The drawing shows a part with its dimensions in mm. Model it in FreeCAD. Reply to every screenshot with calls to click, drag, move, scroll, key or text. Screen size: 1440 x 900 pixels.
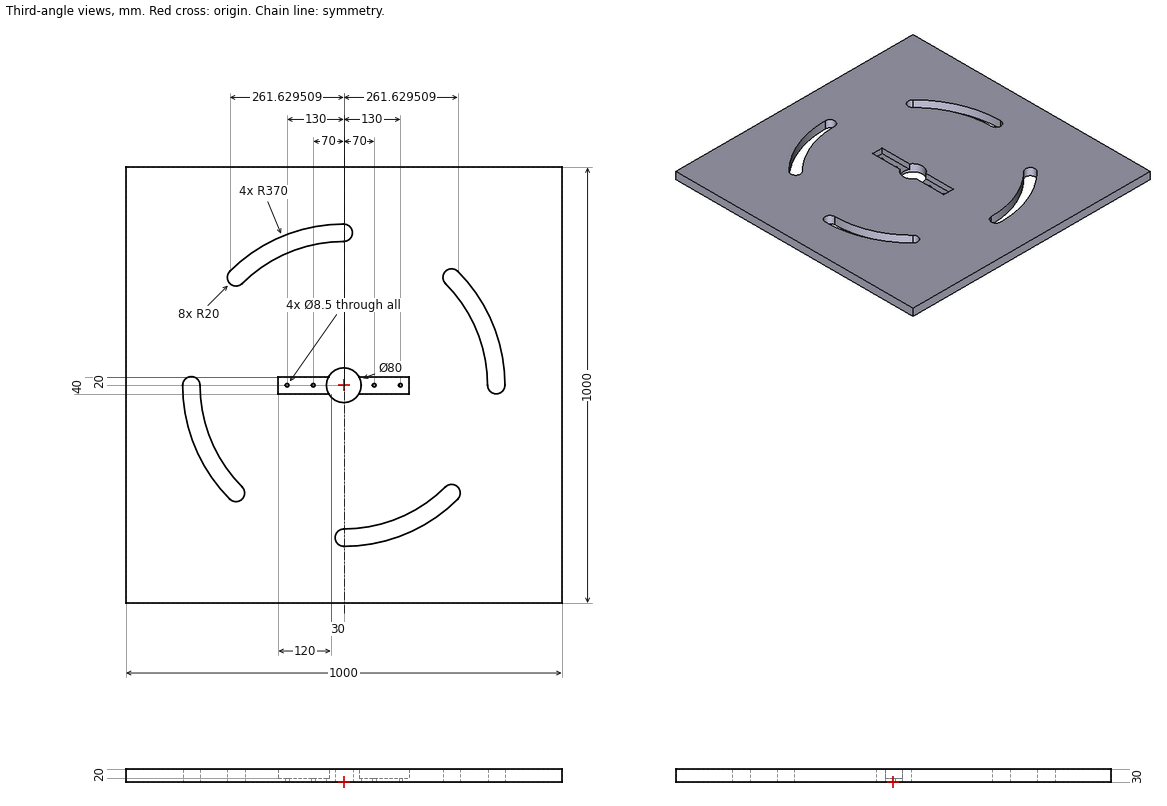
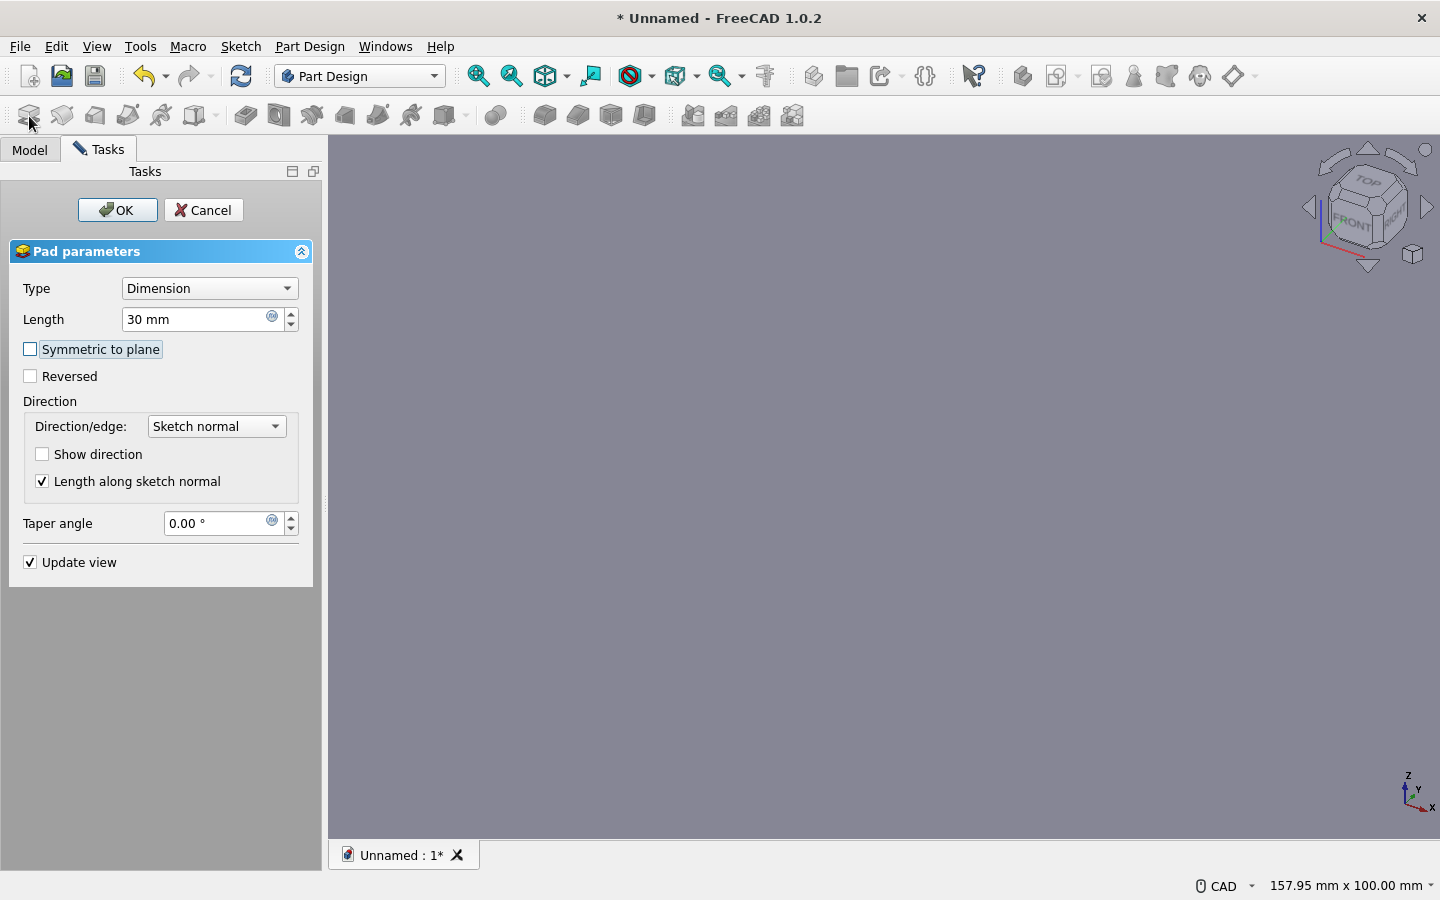
click(118, 210)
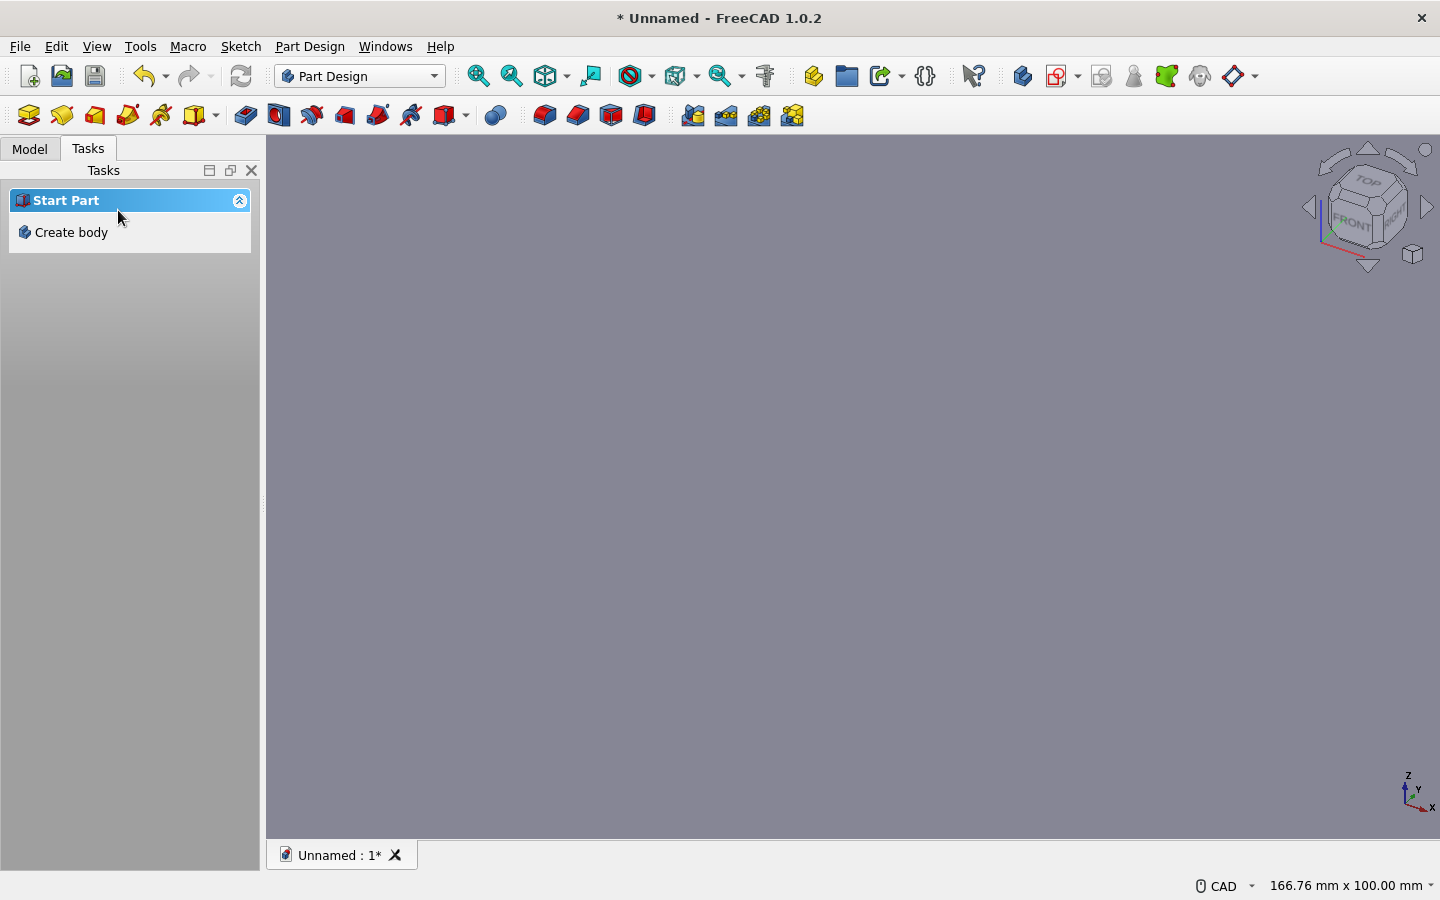
key(v)
key(f)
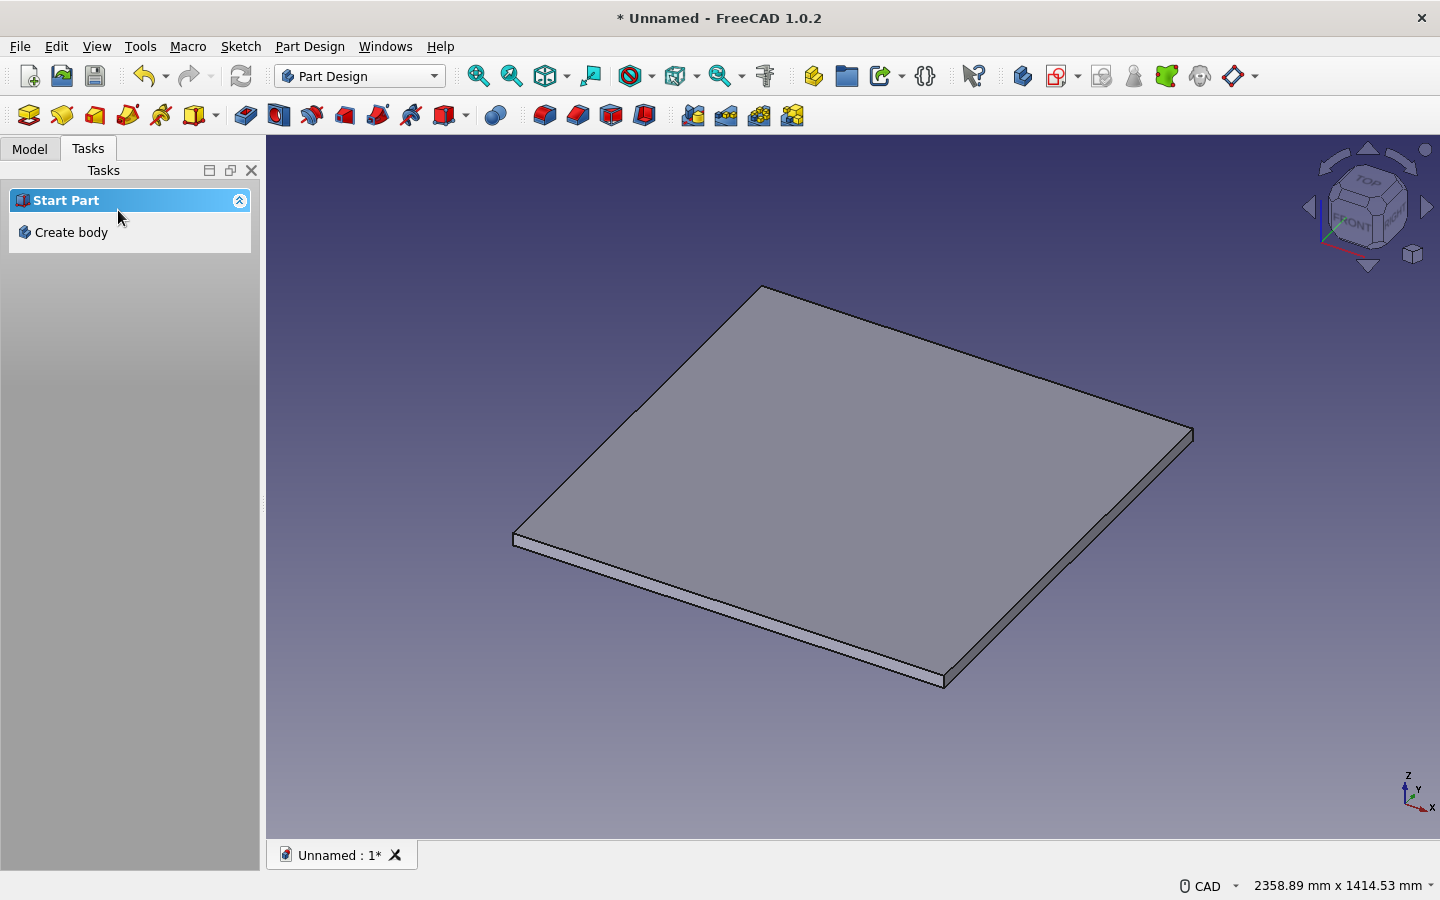
click(853, 480)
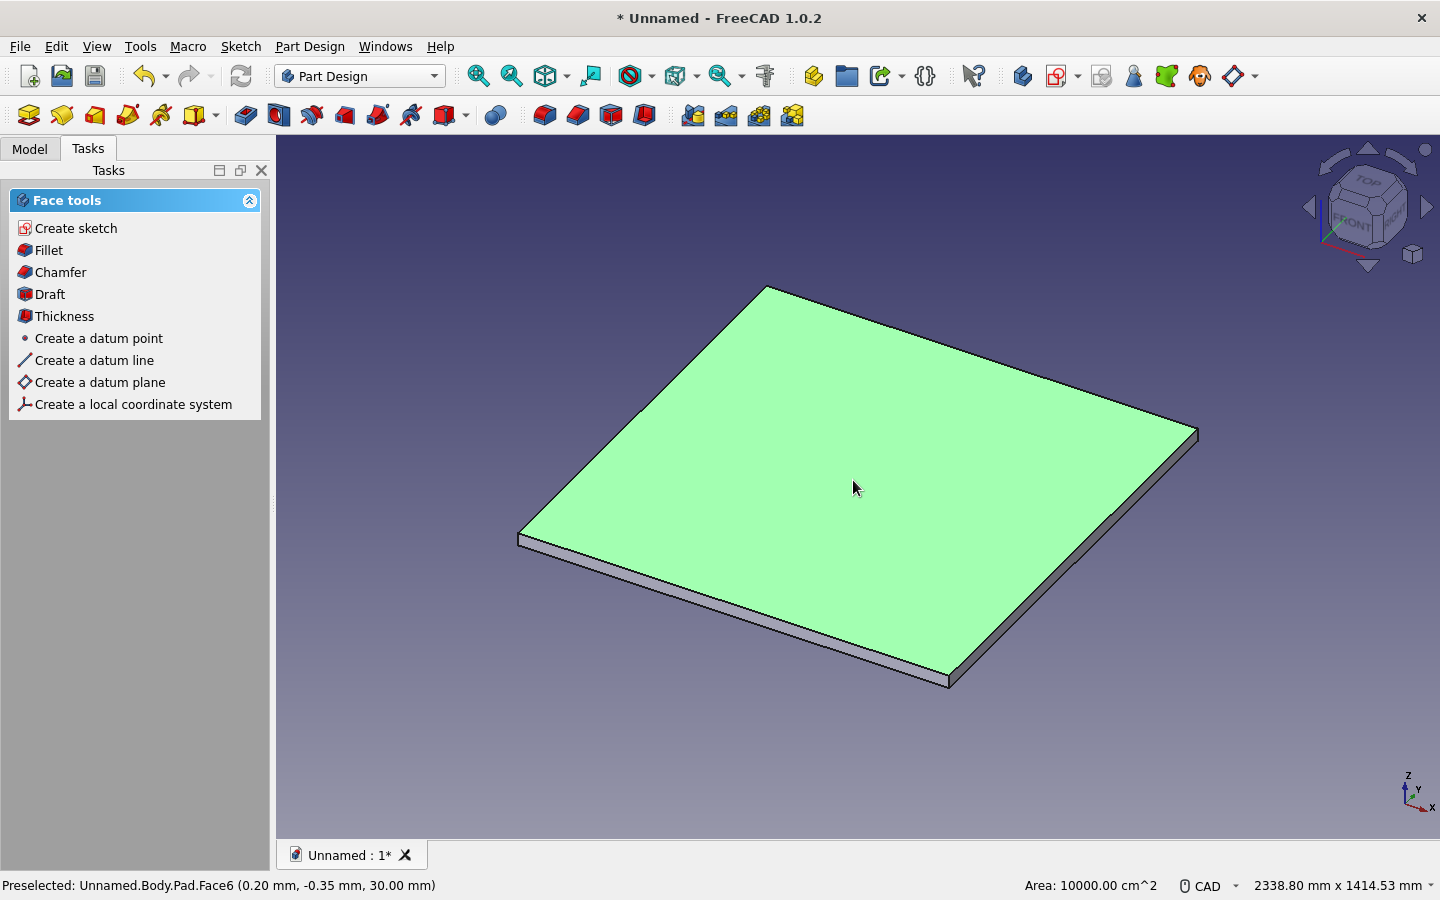
click(1056, 76)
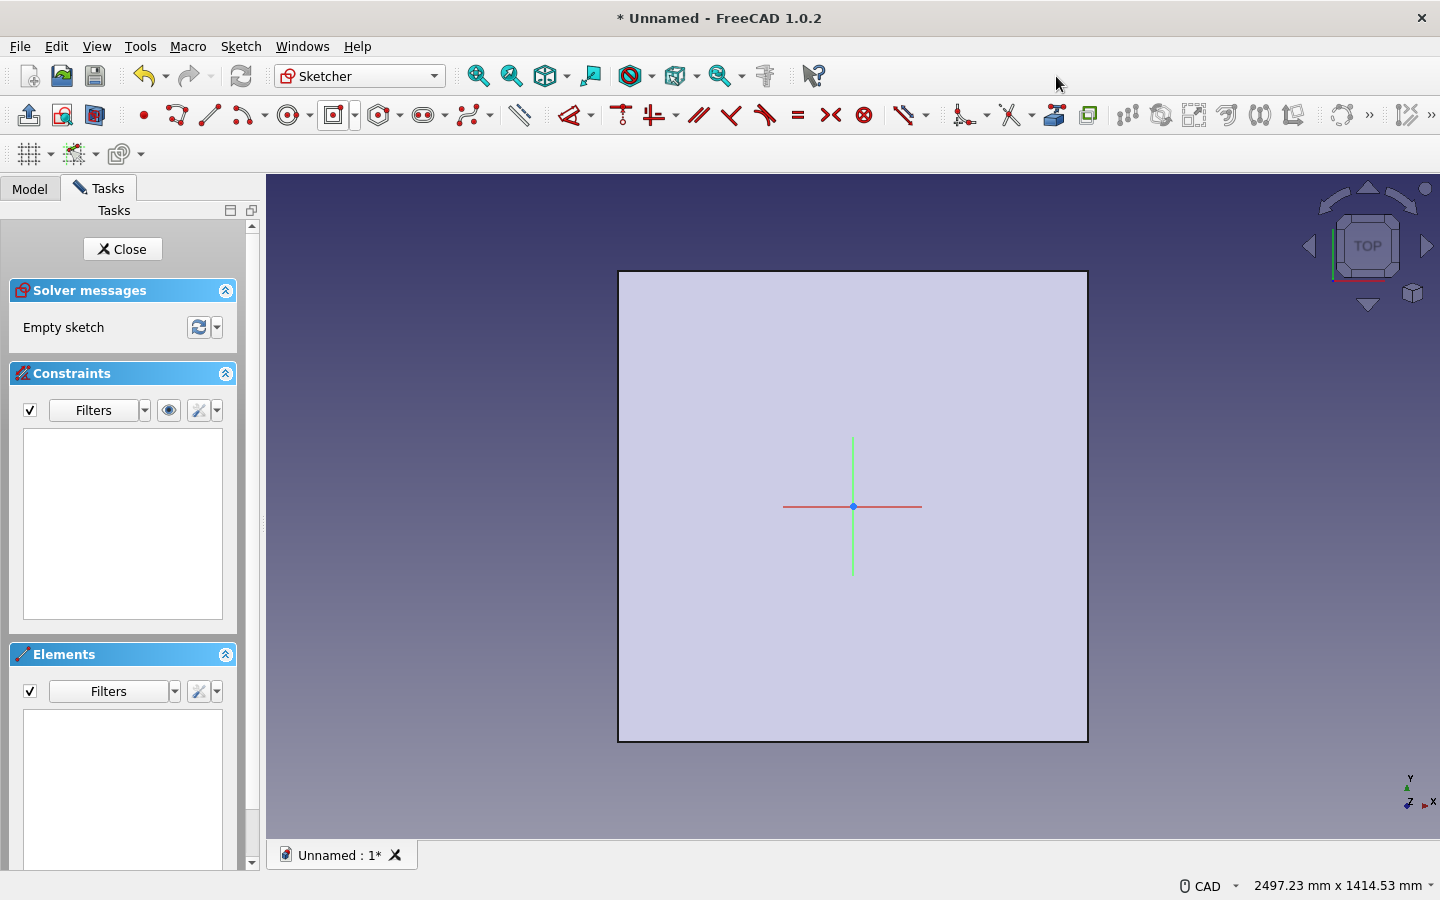
key(g)
key(3)
key(a)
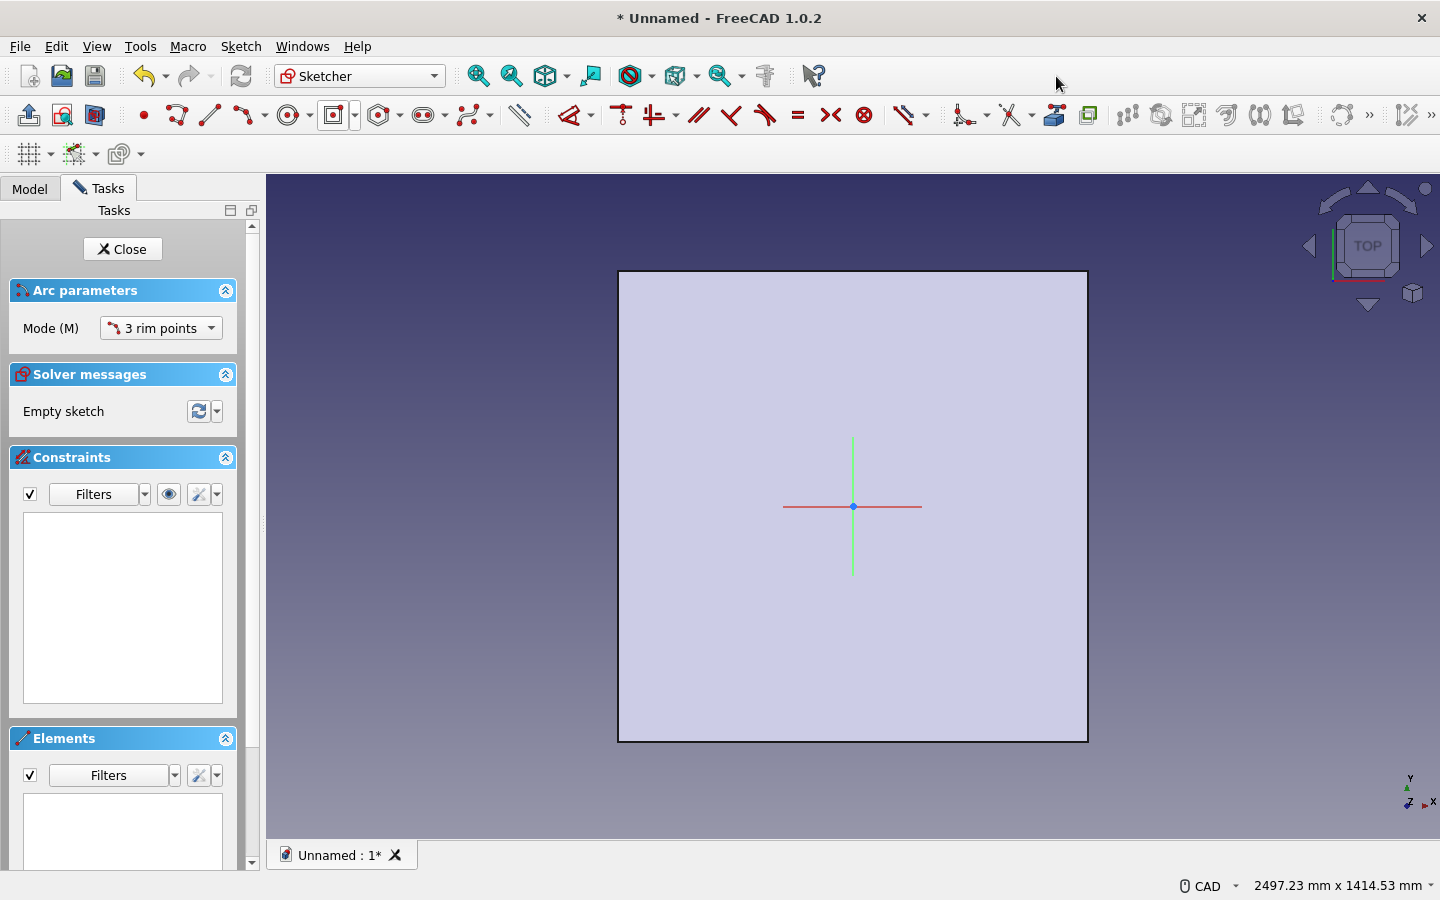
click(853, 351)
click(853, 333)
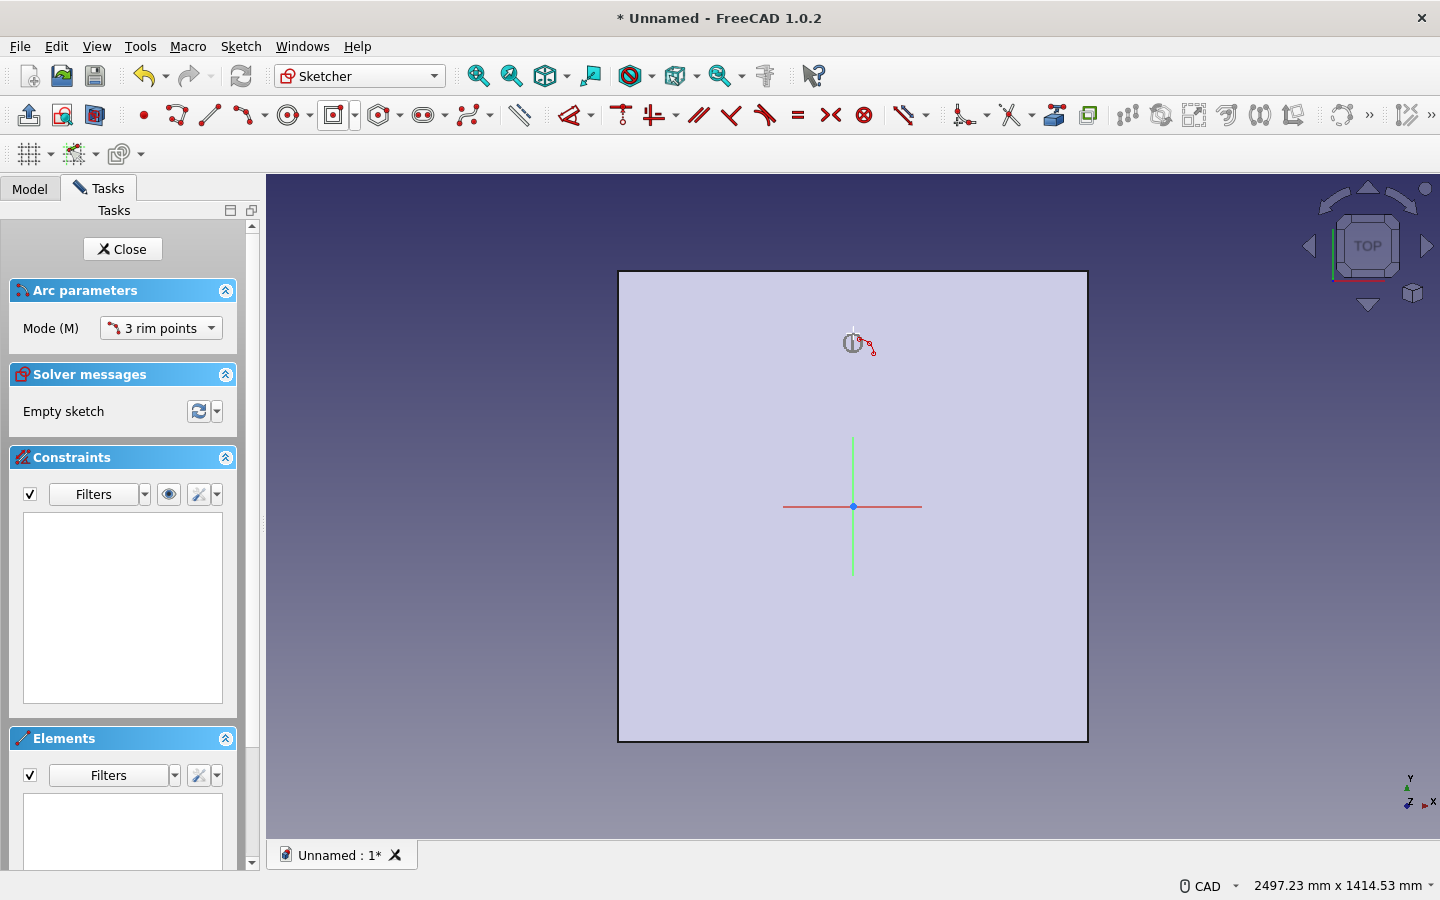
scroll(862, 342, up, 3)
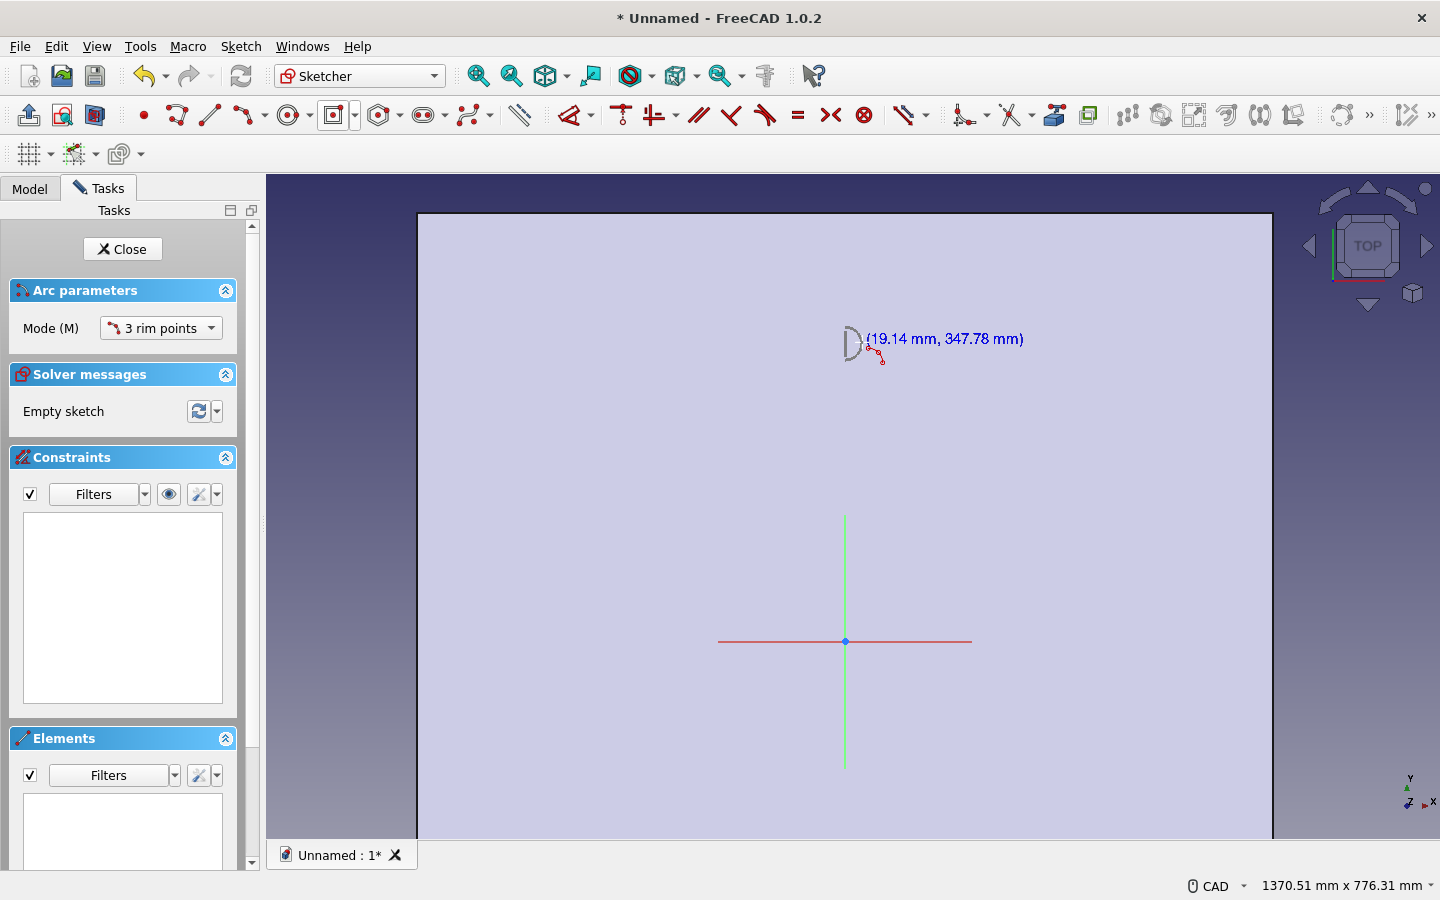
click(862, 342)